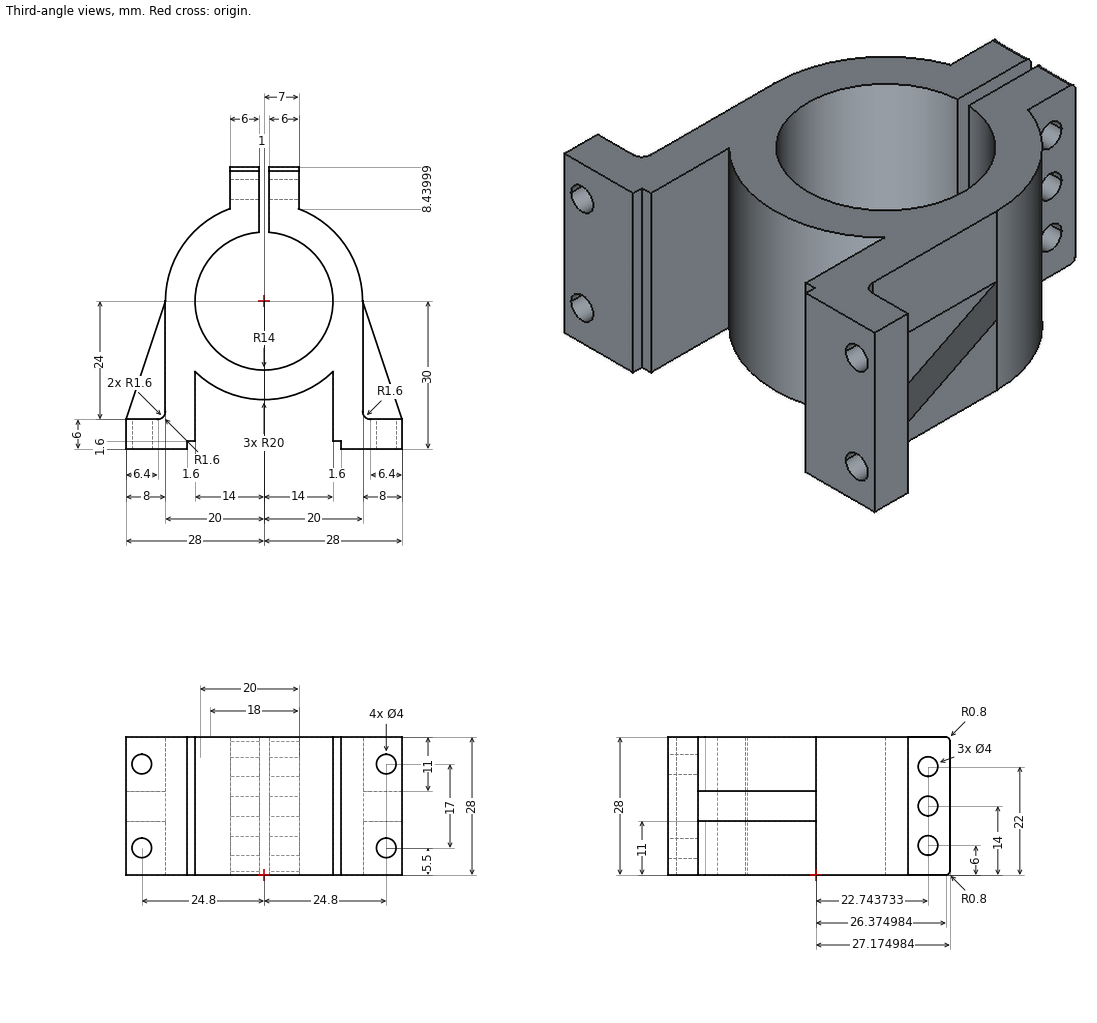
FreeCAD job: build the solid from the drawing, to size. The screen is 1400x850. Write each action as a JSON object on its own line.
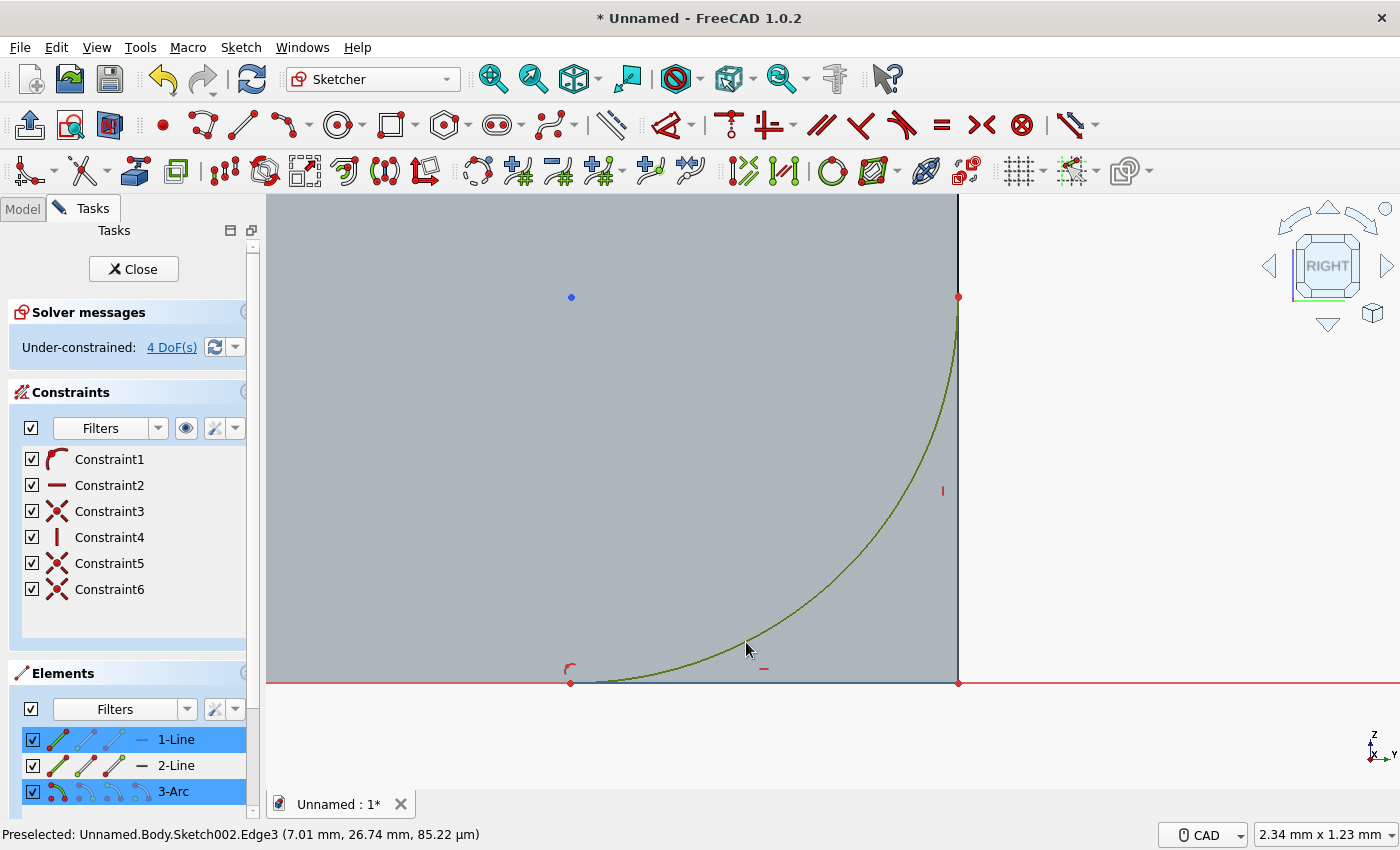
{"action": "left_click", "coordinate": [902, 126]}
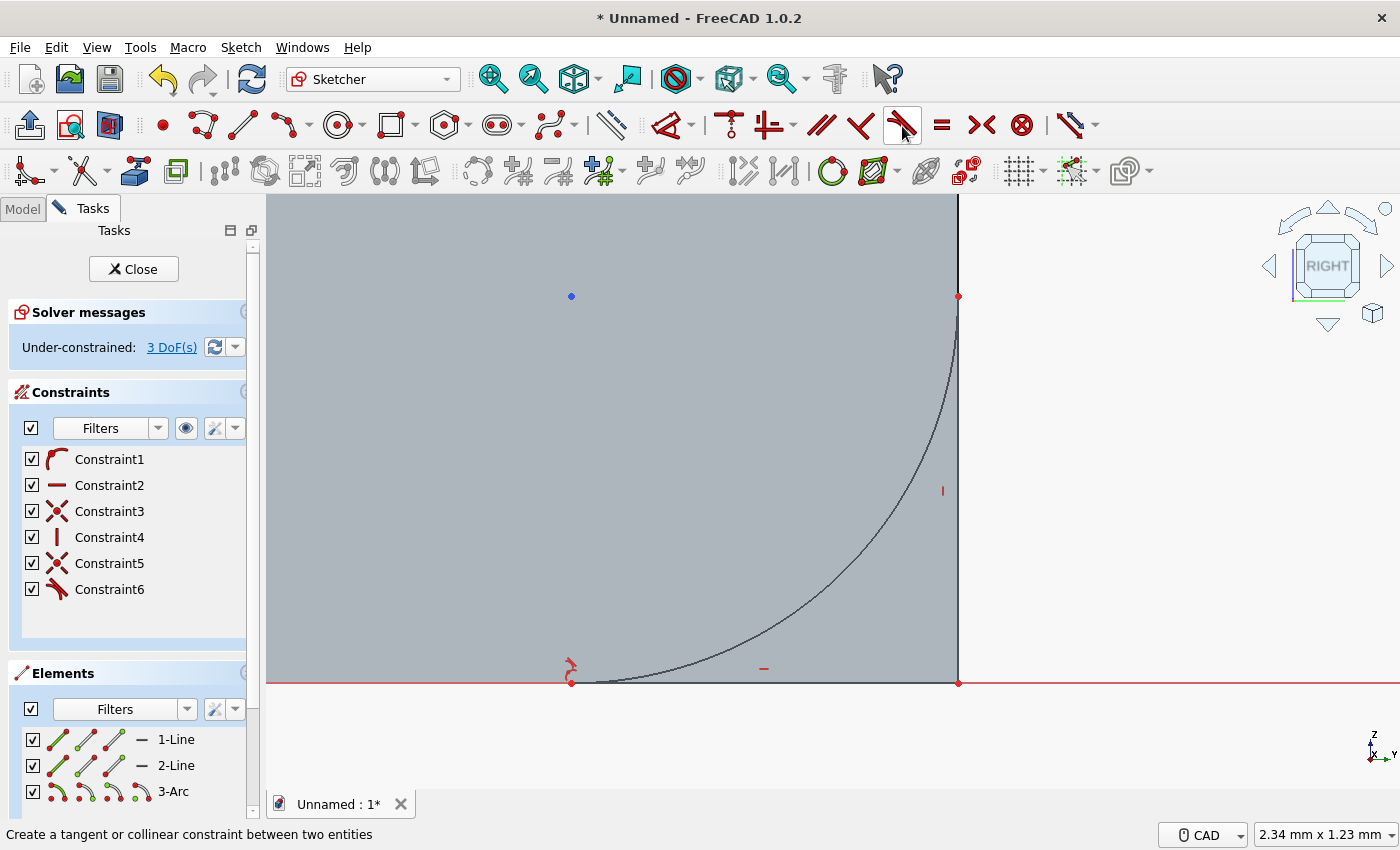
{"action": "left_click", "coordinate": [958, 567]}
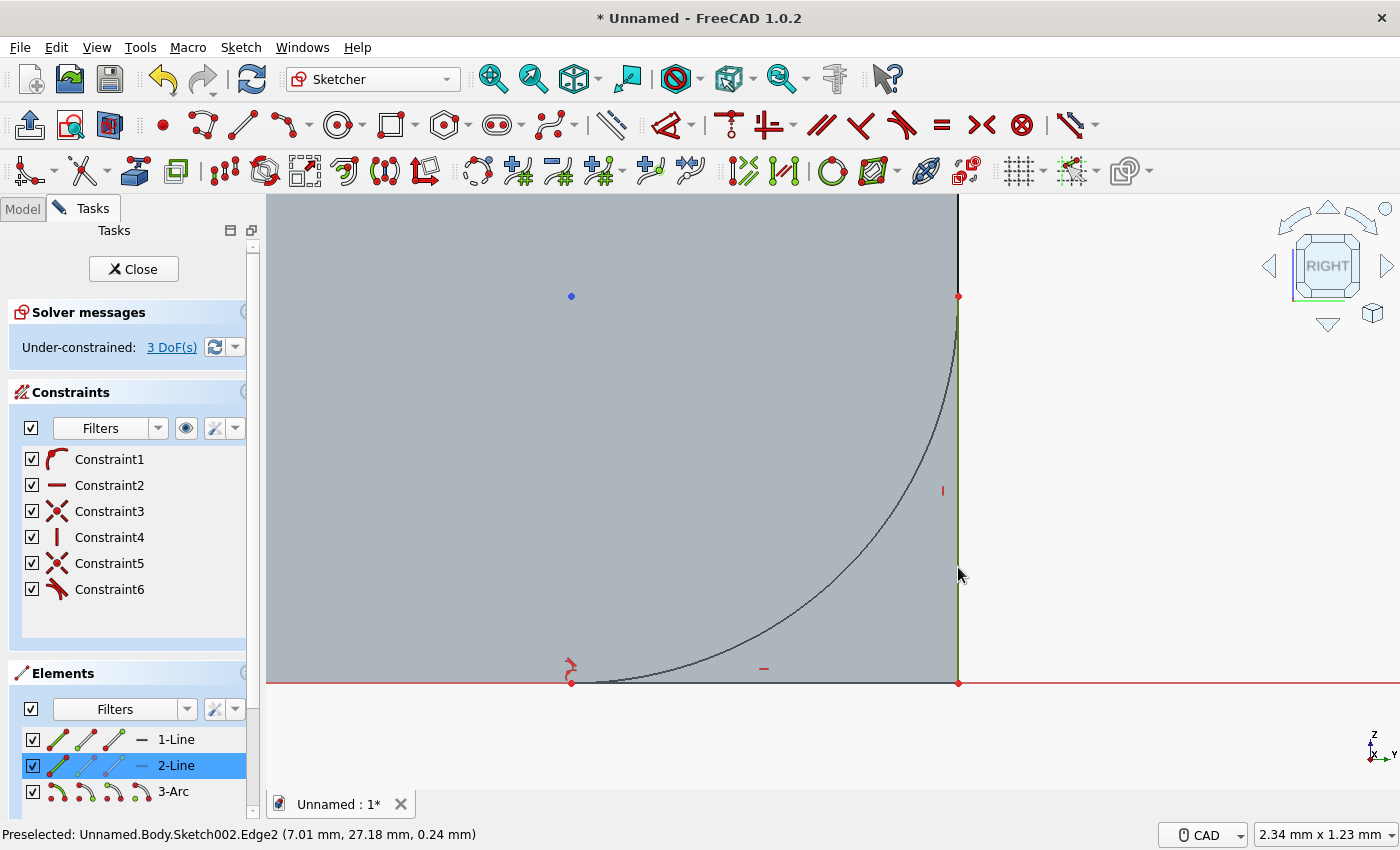
{"action": "left_click", "coordinate": [747, 641]}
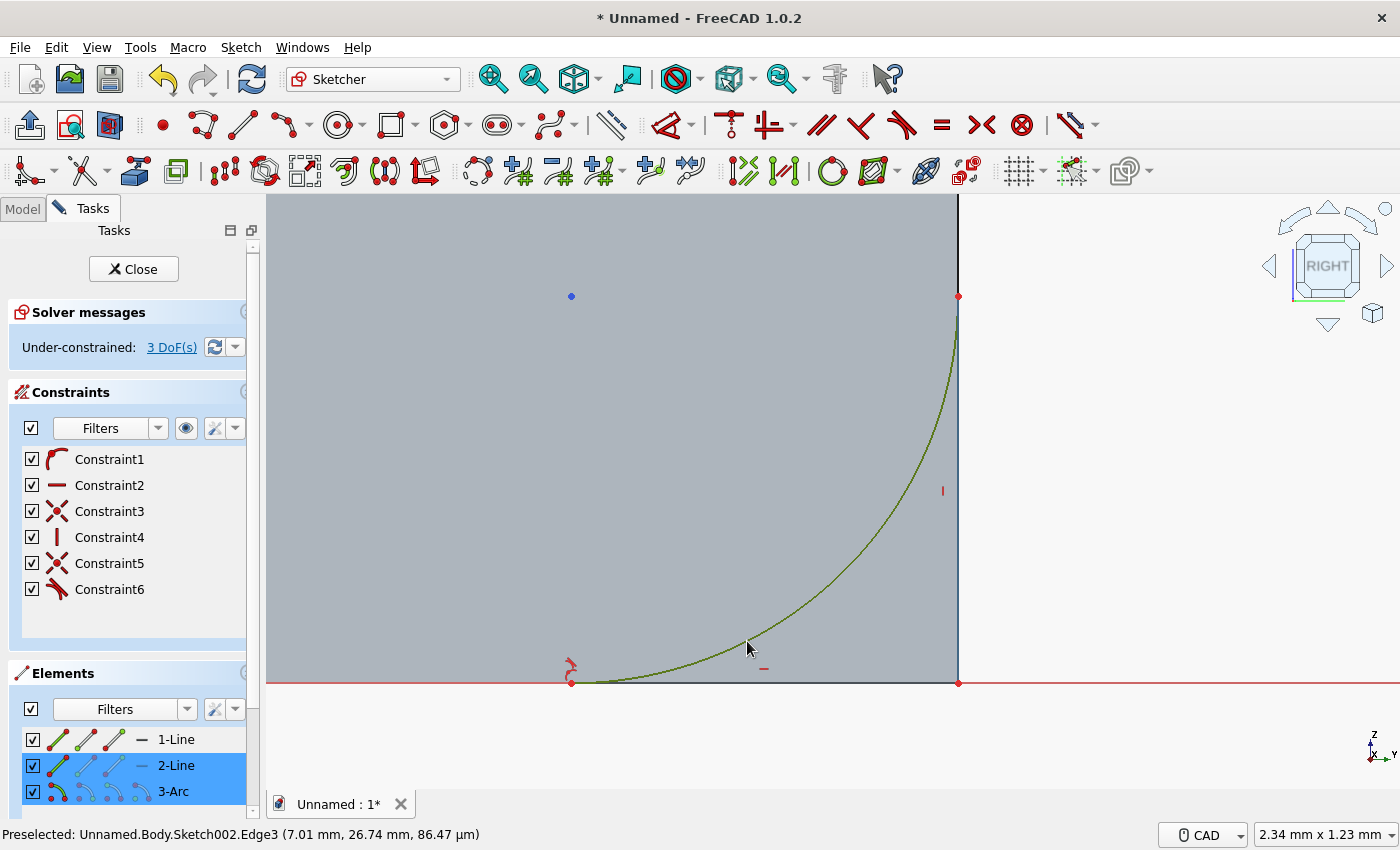
{"action": "left_click", "coordinate": [902, 126]}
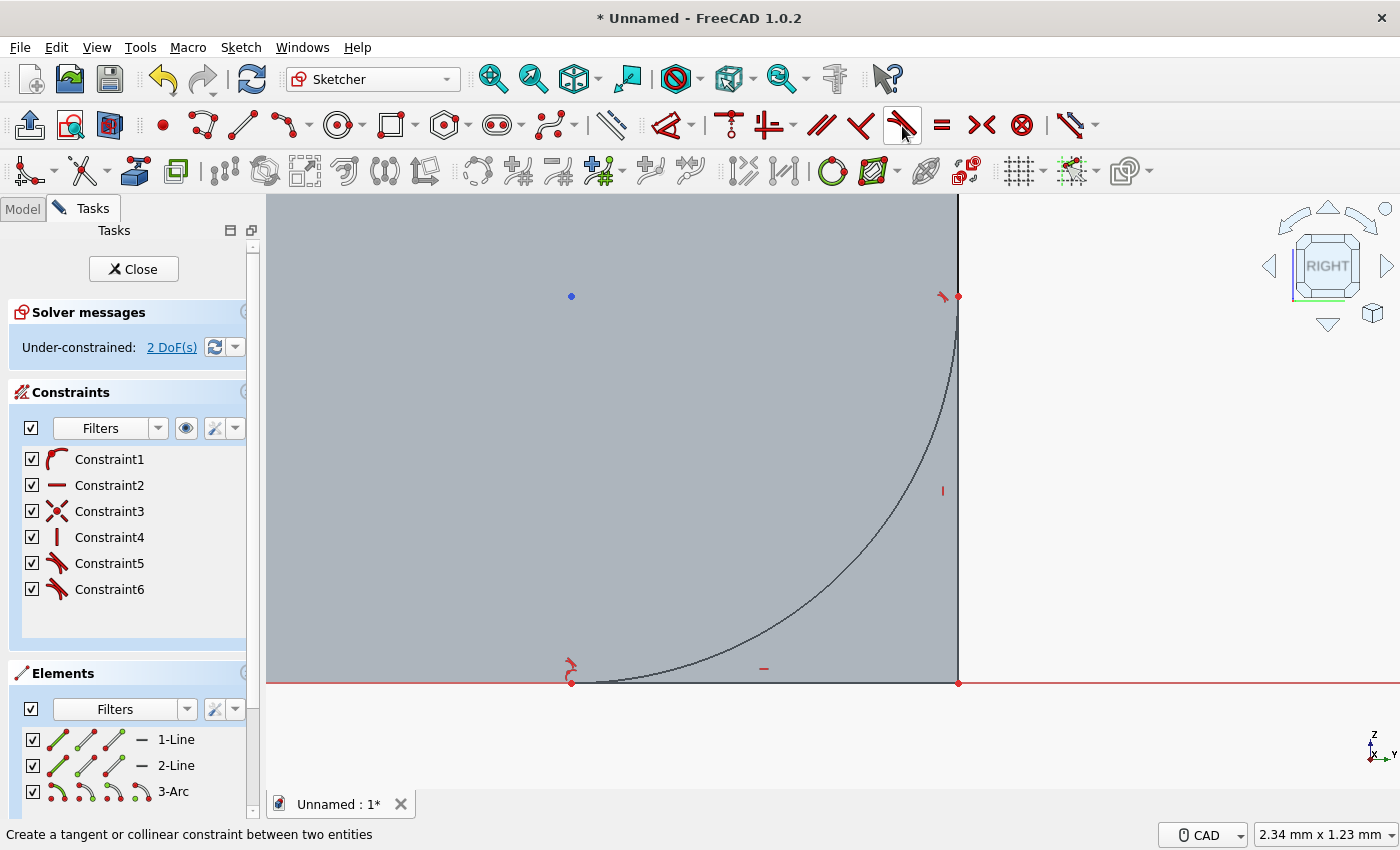
{"action": "left_click", "coordinate": [666, 126]}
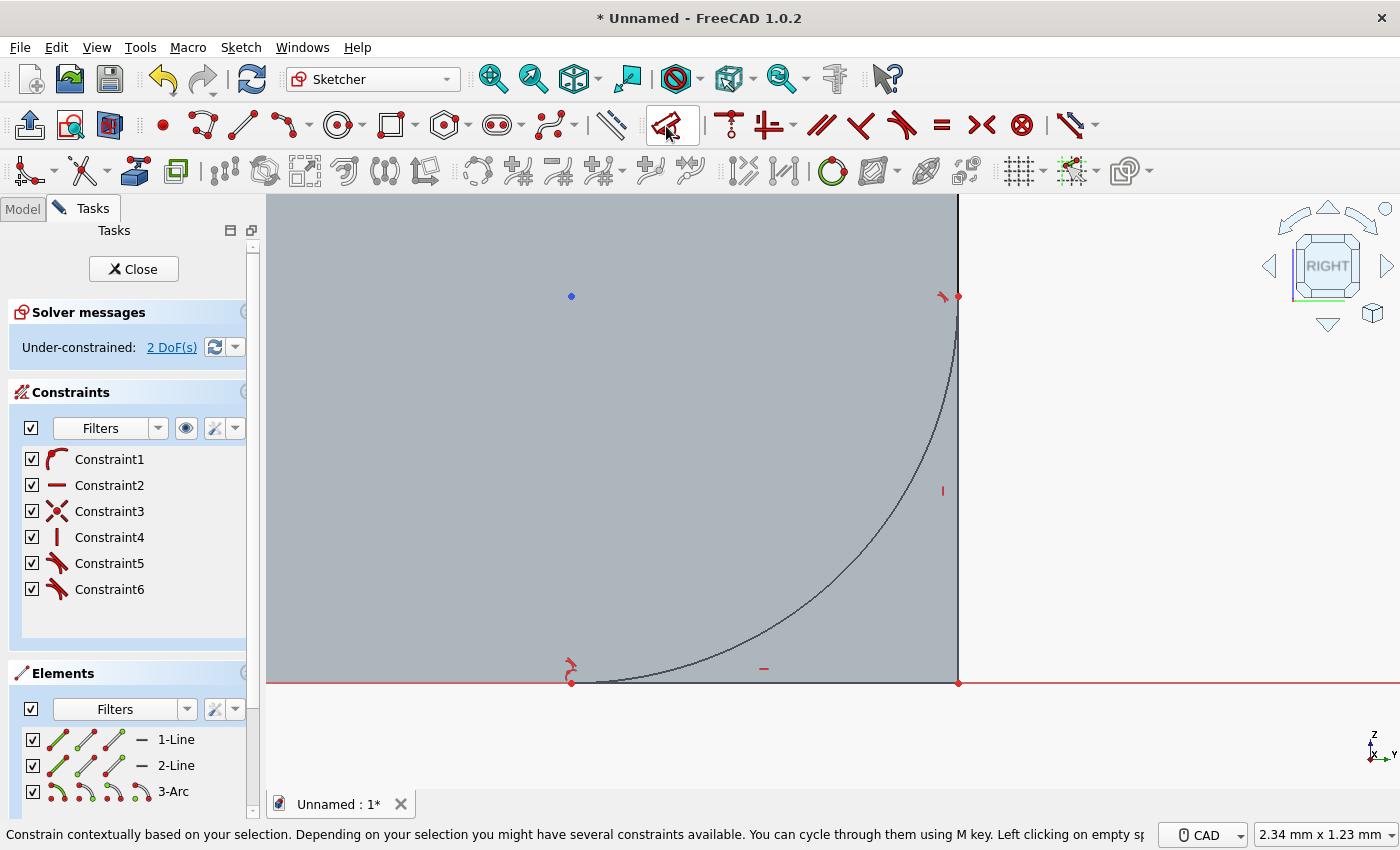
{"action": "left_click", "coordinate": [747, 641]}
{"action": "left_click", "coordinate": [762, 670]}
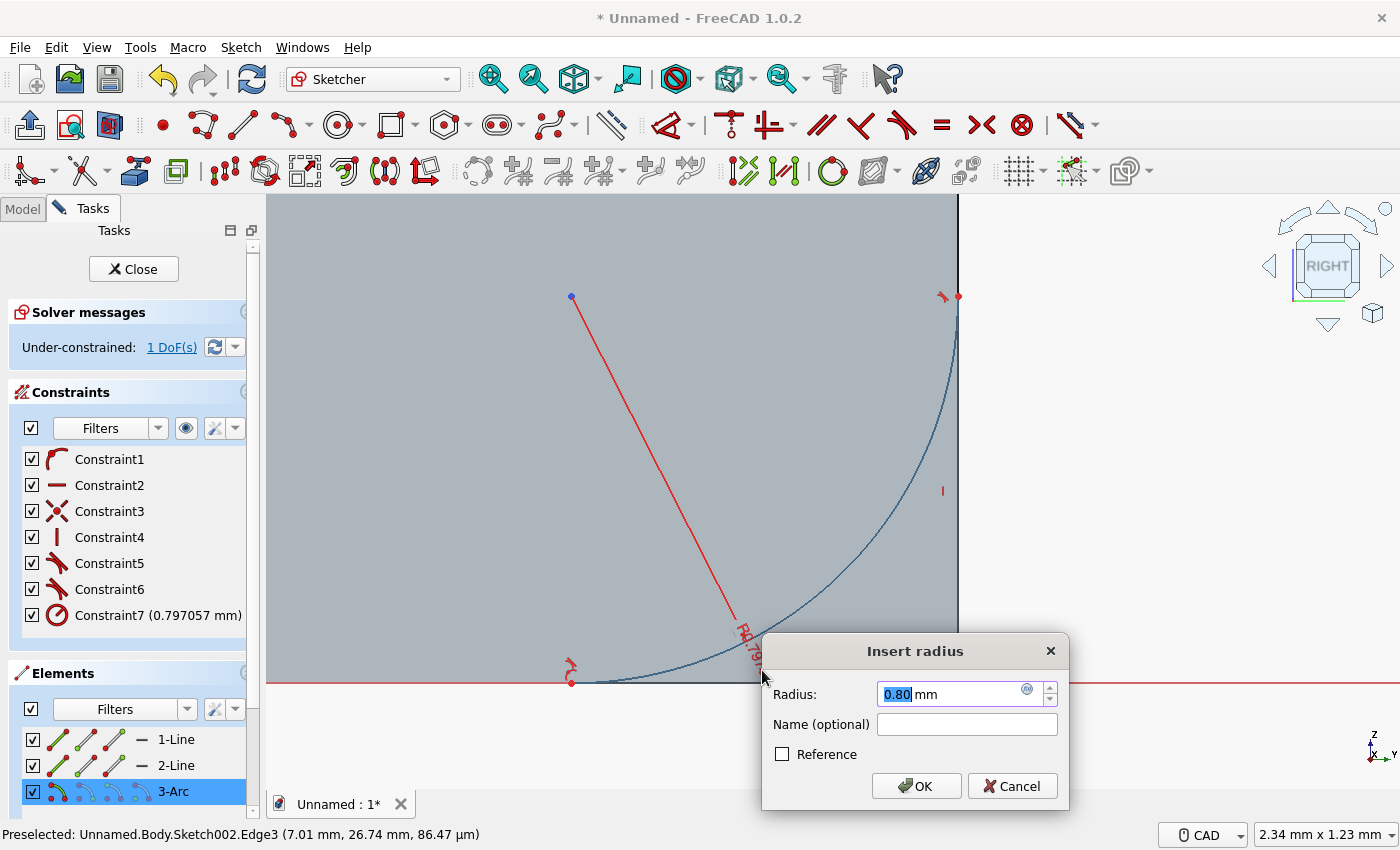
{"action": "type", "text": "0.8"}
{"action": "key", "text": "Return"}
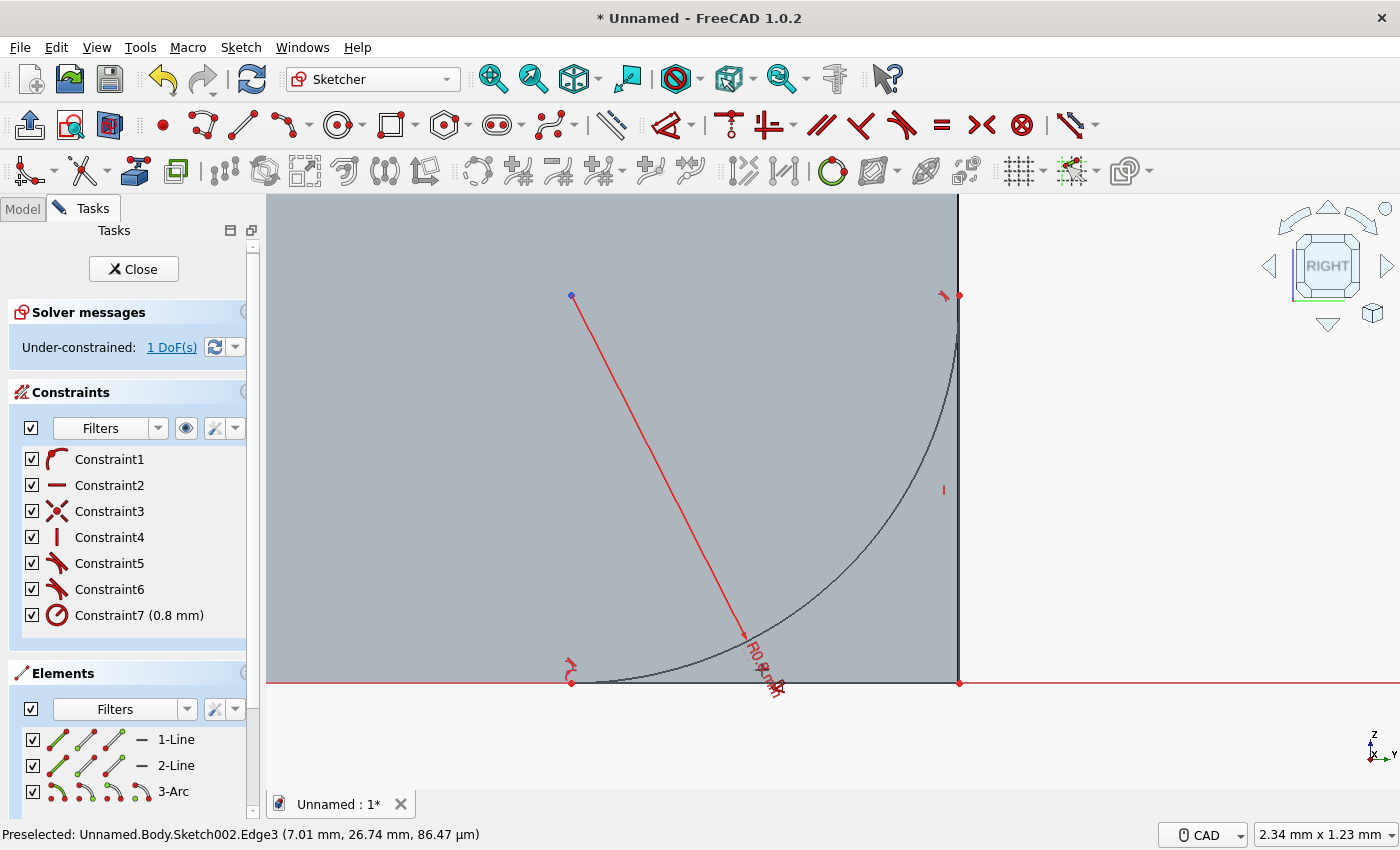
{"action": "left_click", "coordinate": [572, 683]}
{"action": "left_click", "coordinate": [433, 717]}